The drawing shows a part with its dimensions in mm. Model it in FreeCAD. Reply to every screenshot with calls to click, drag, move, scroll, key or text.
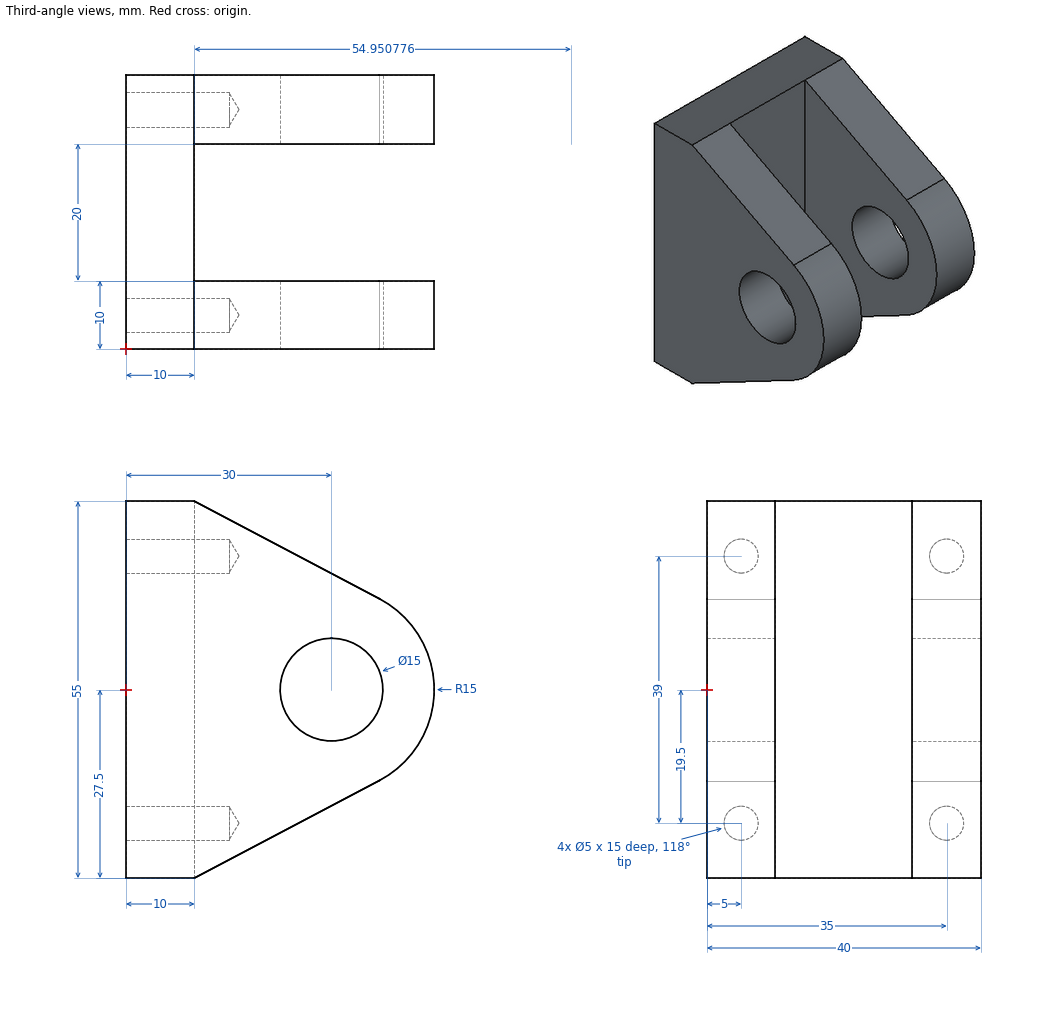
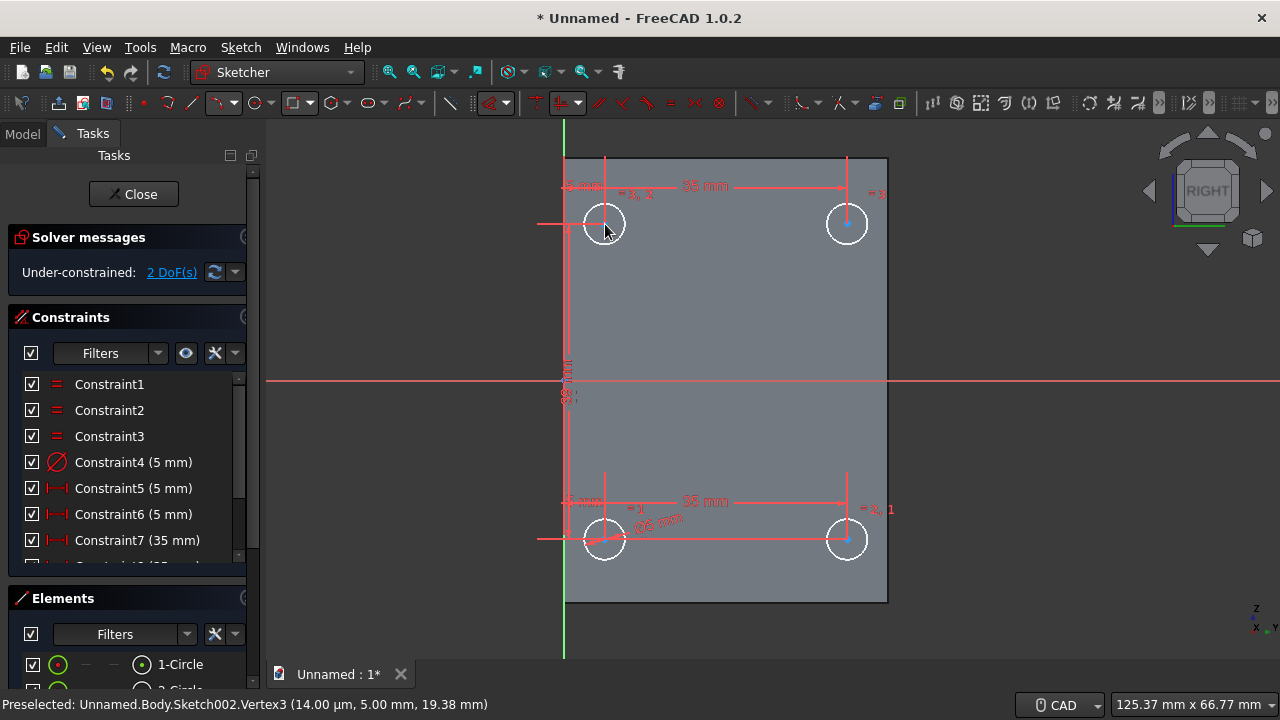
click(847, 539)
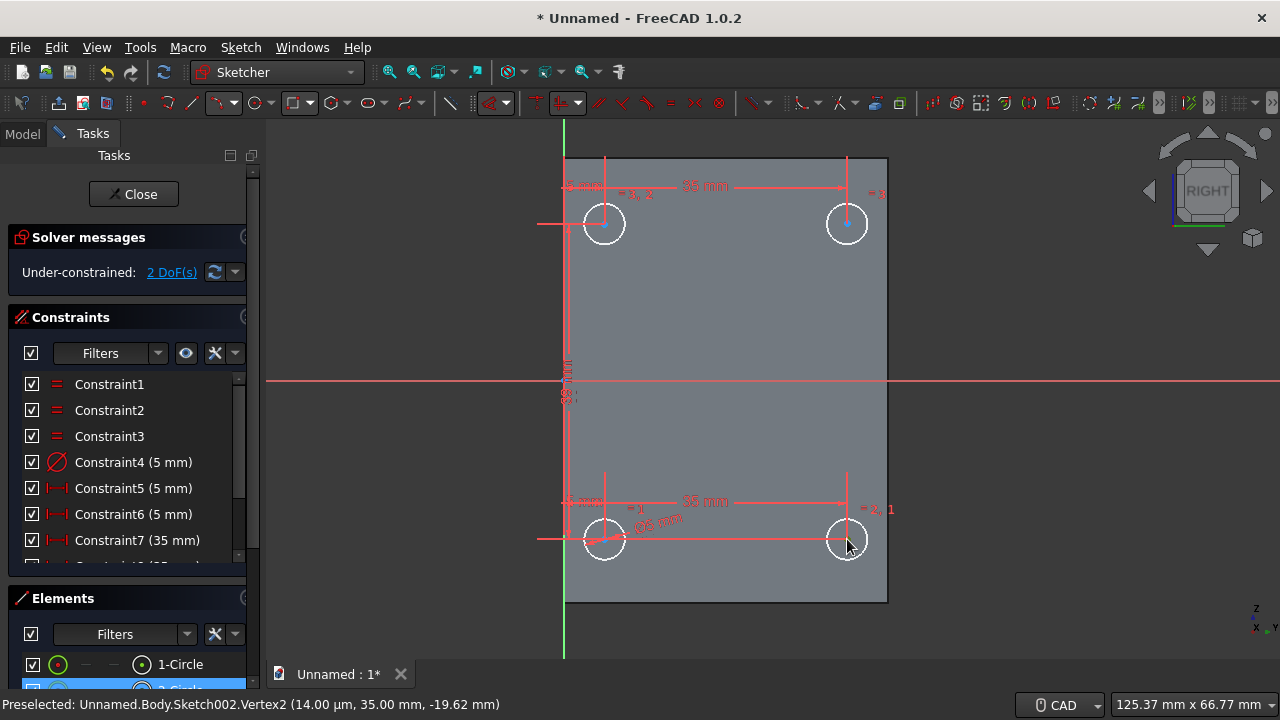
click(847, 224)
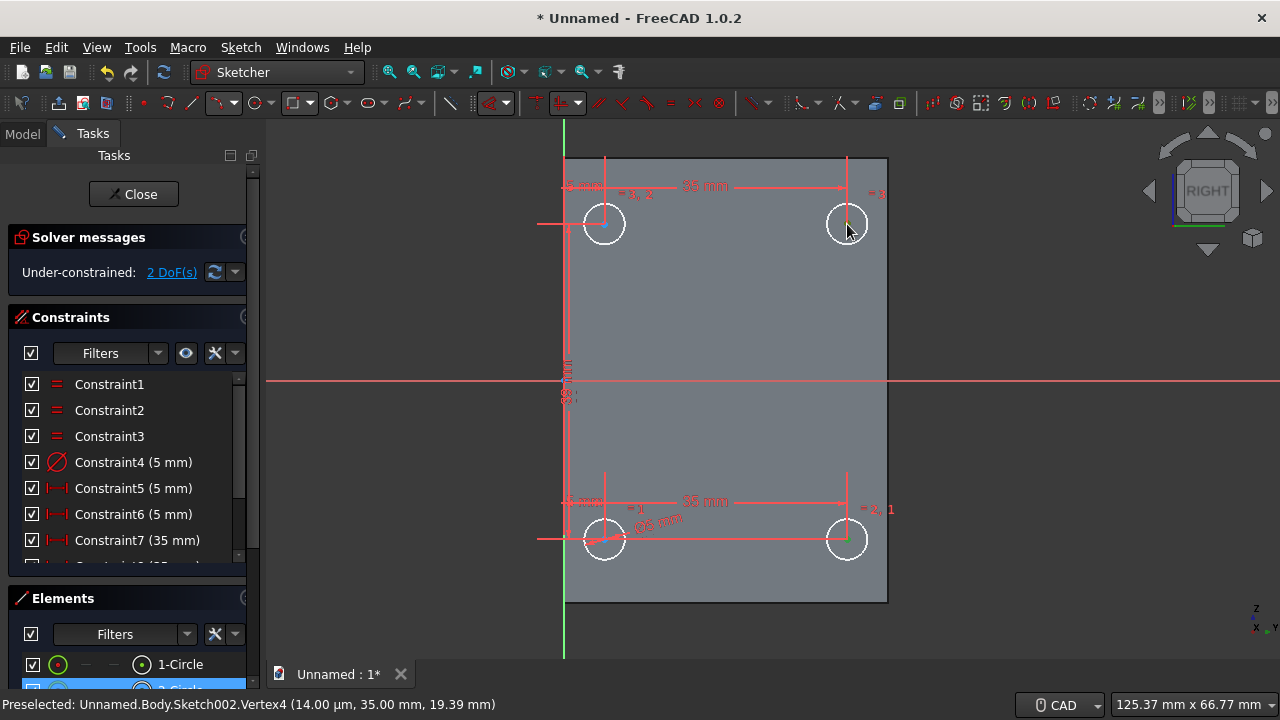
key(i)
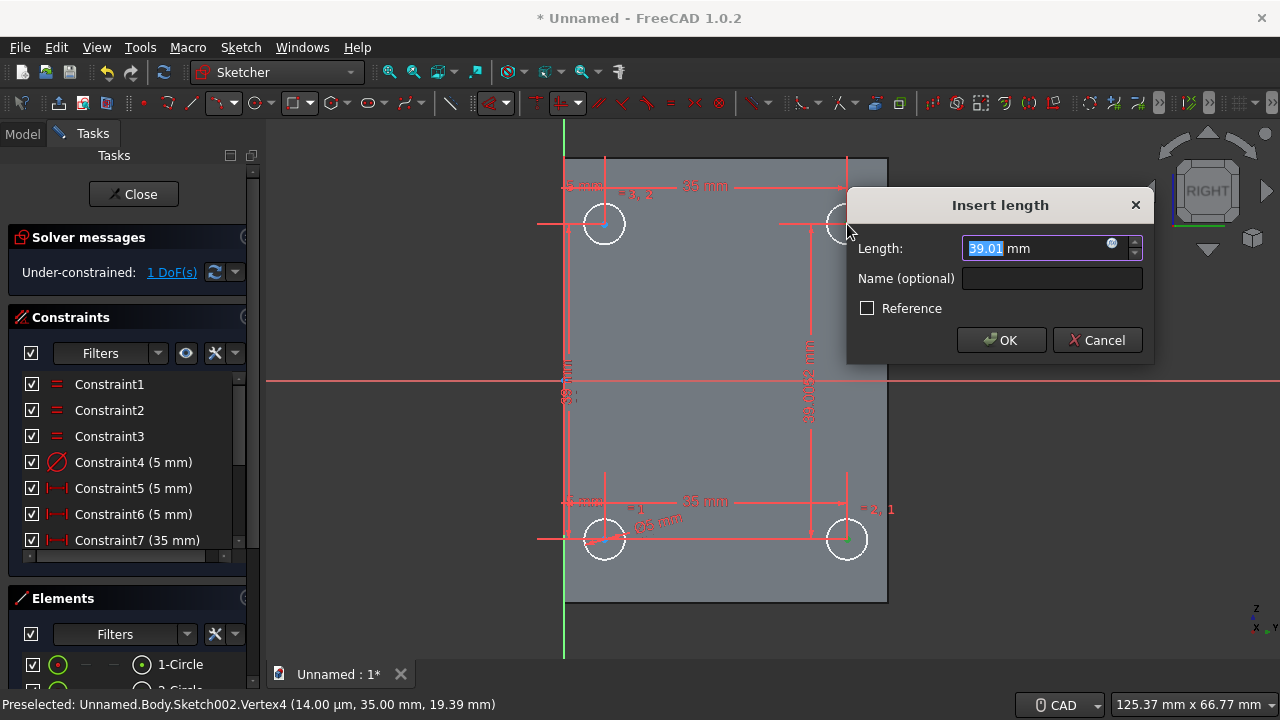
text(39)
key(Return)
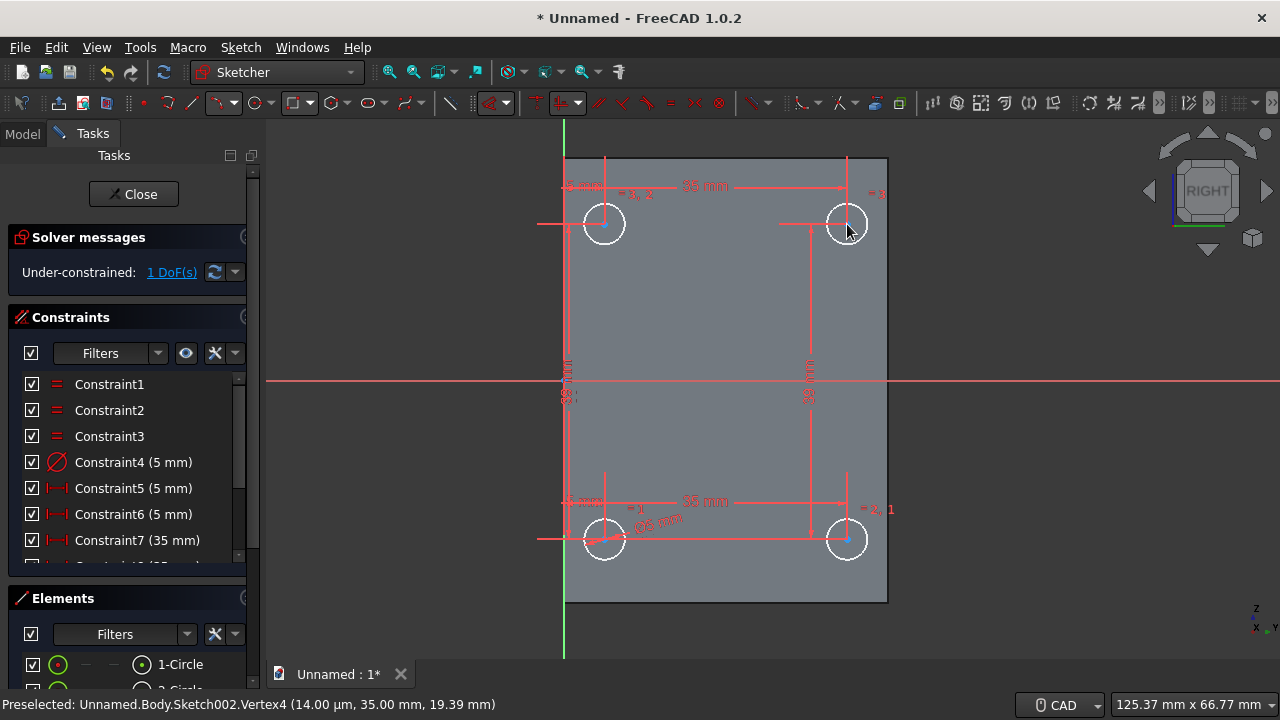
click(605, 539)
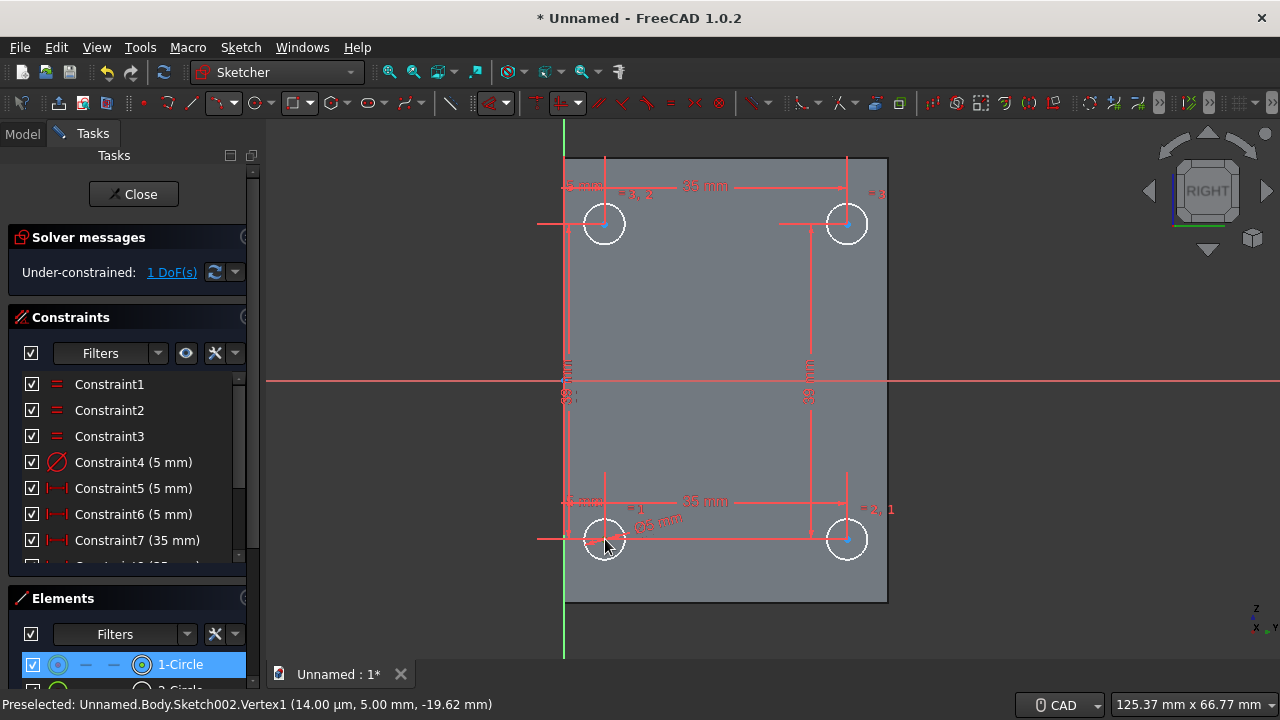
key(i)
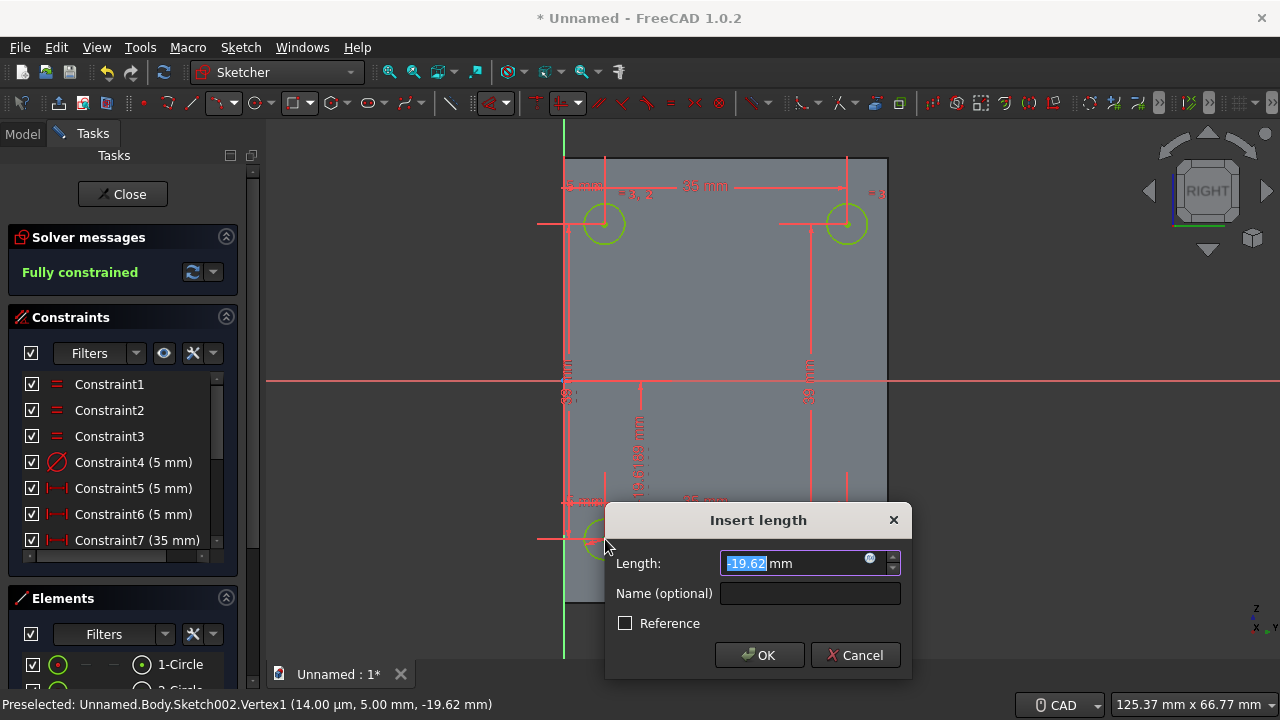
text(-19.5)
key(Return)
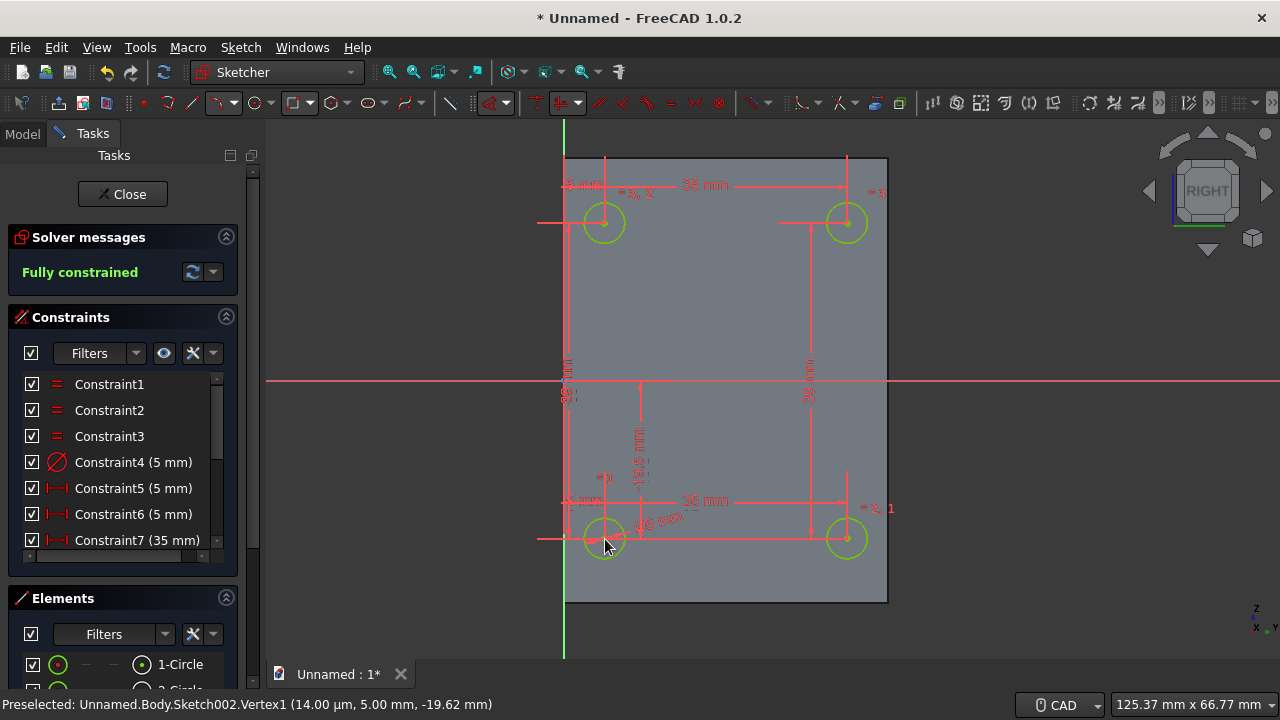
click(123, 194)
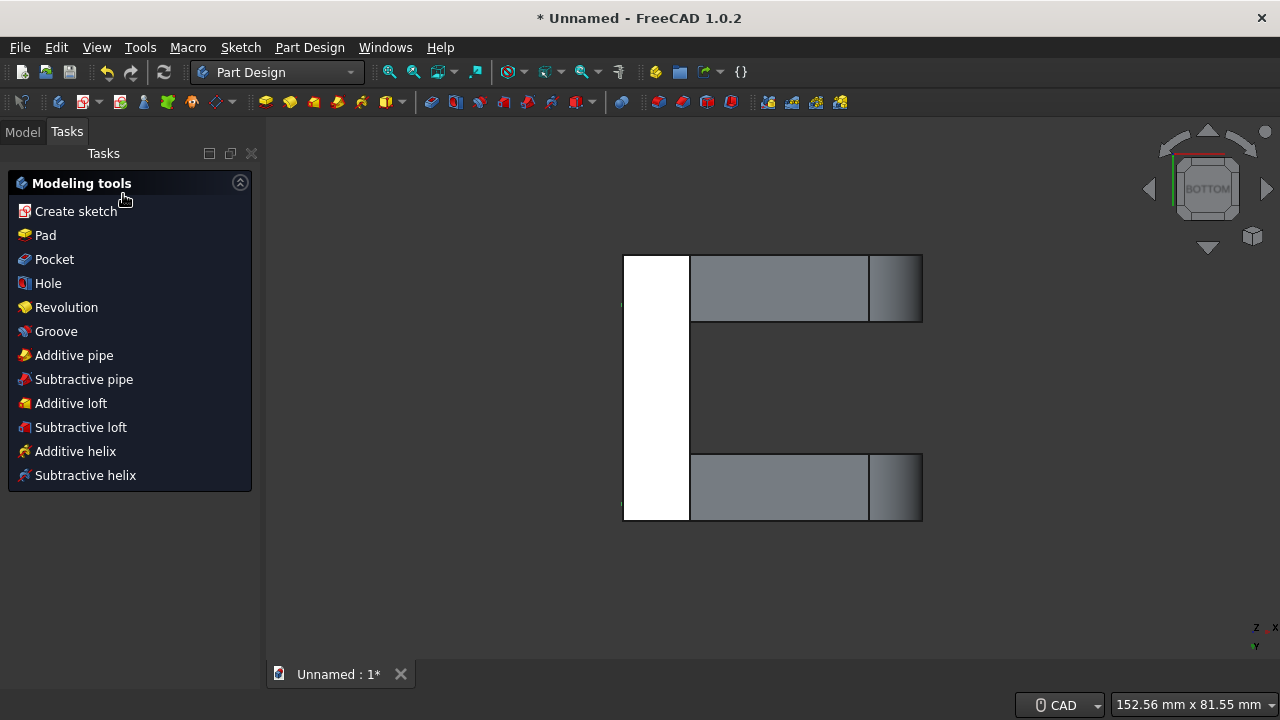
click(456, 102)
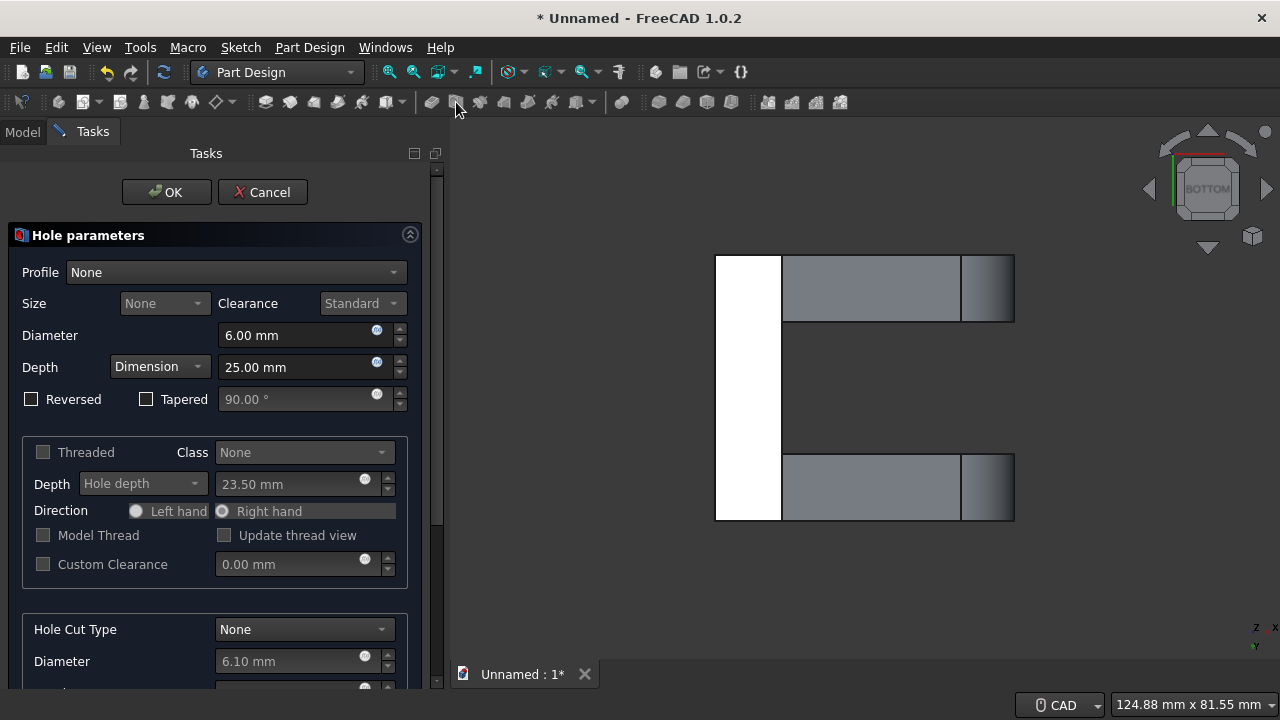
triple_click(305, 335)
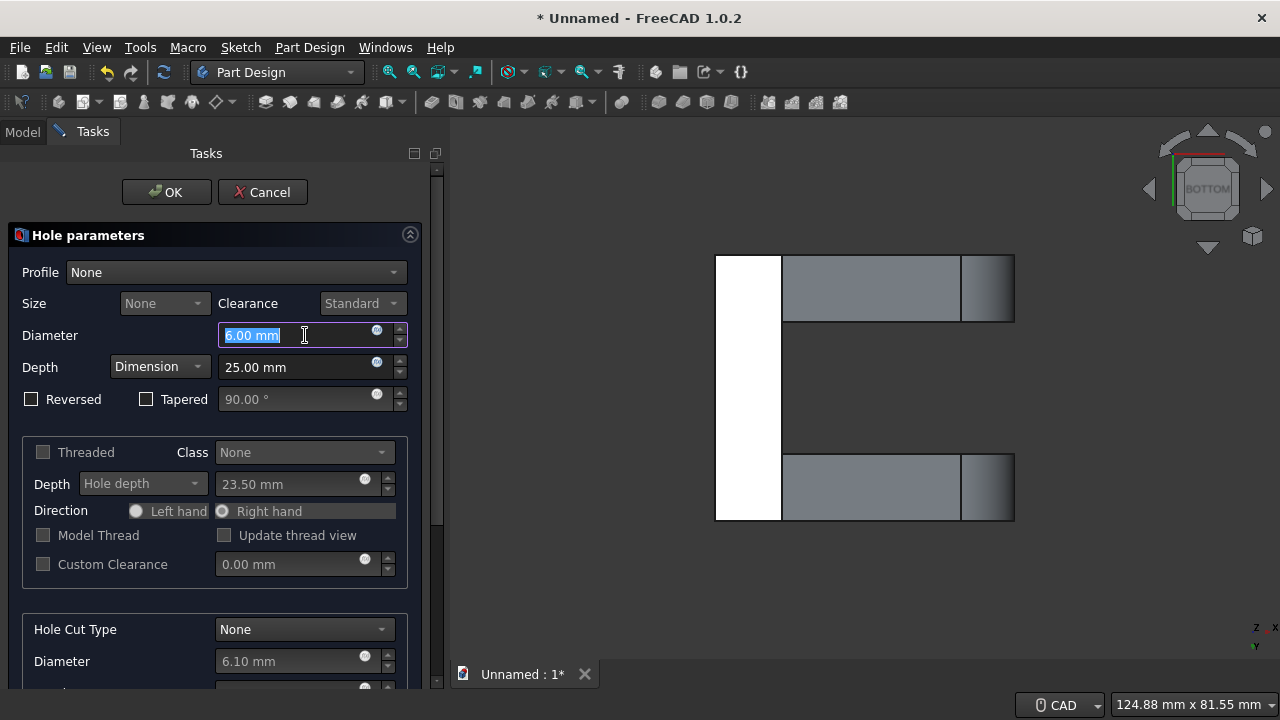
text(5)
key(Tab)